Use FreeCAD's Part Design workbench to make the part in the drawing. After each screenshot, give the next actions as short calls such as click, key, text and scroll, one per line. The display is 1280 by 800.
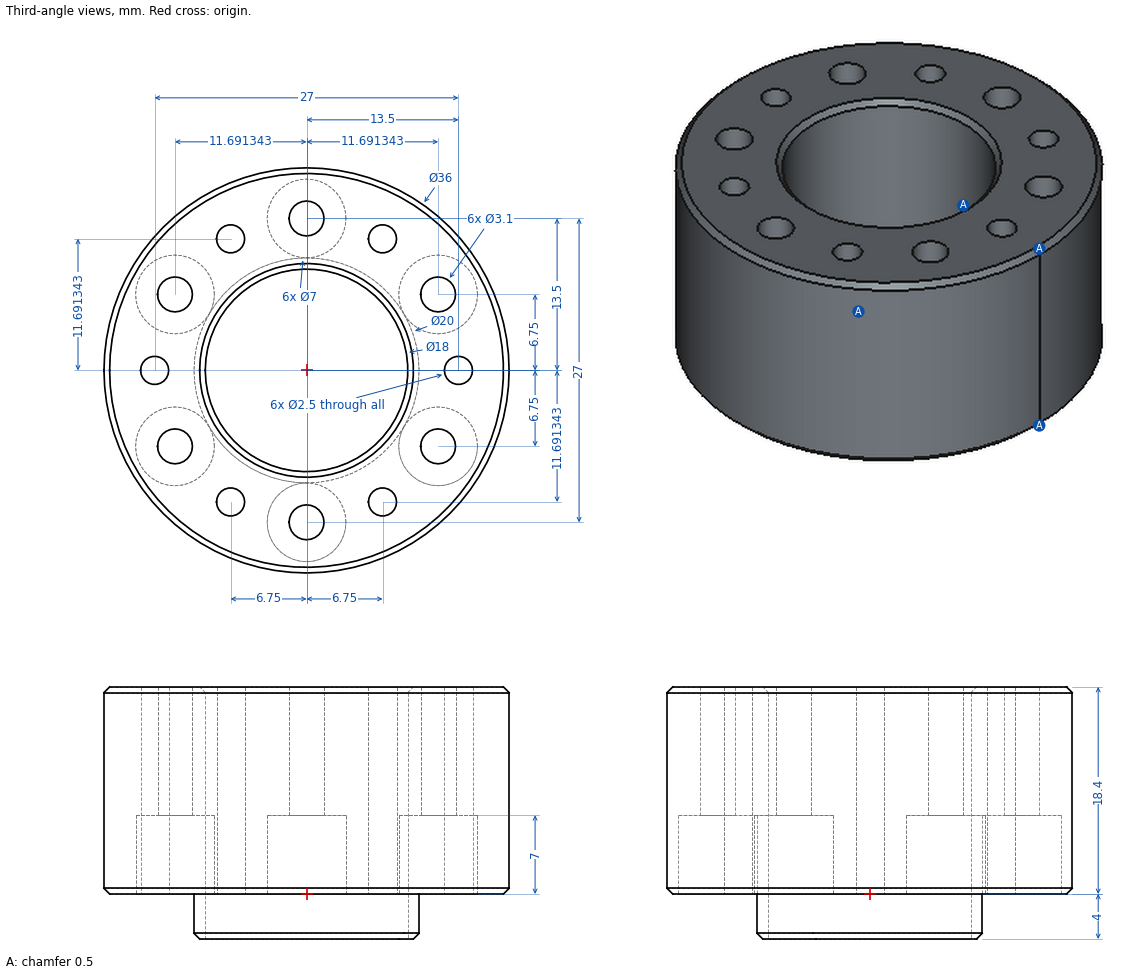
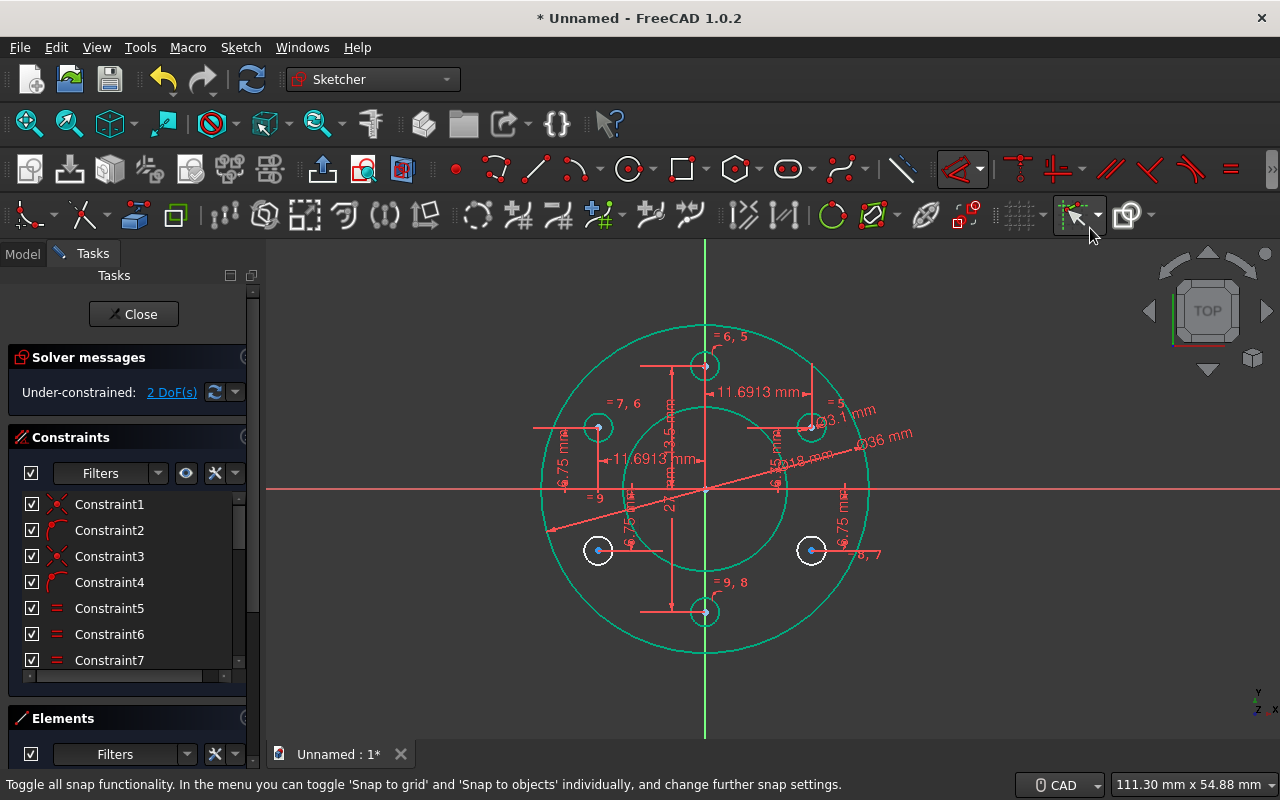
click(812, 551)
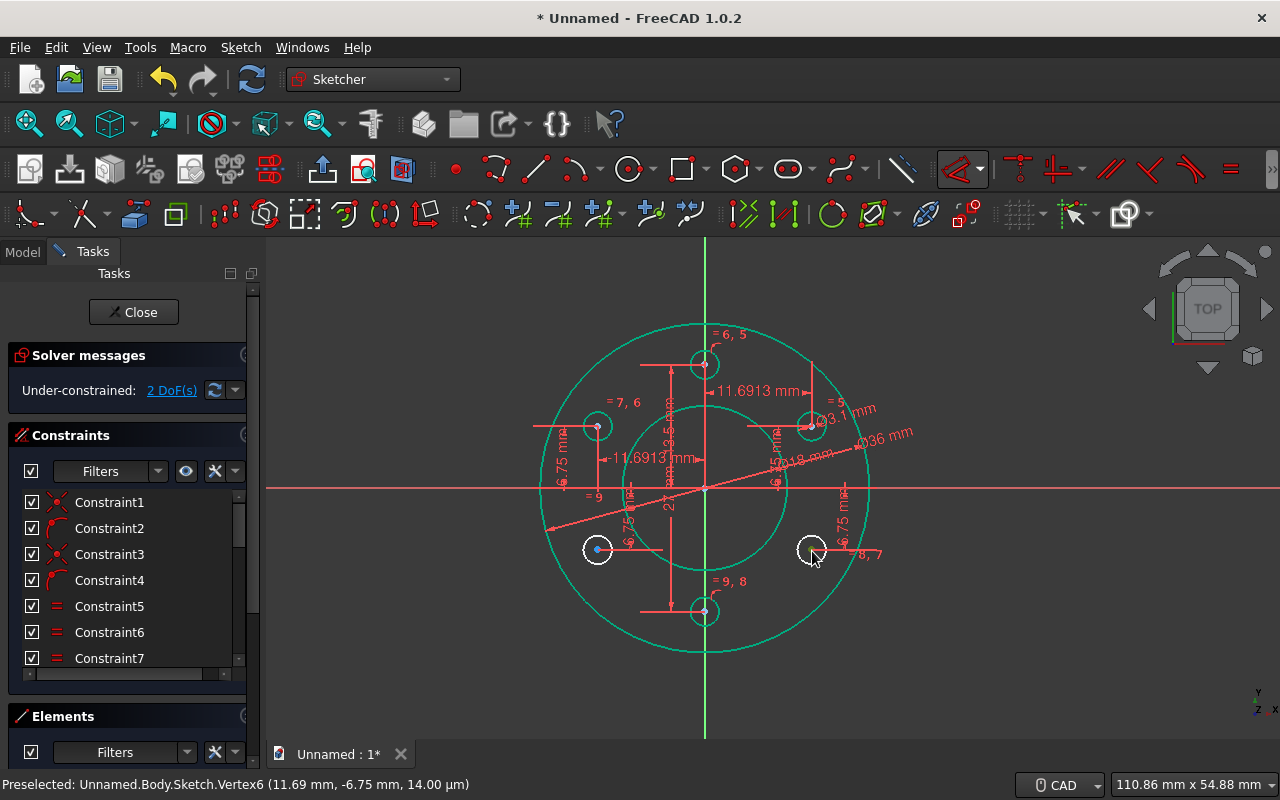
click(982, 170)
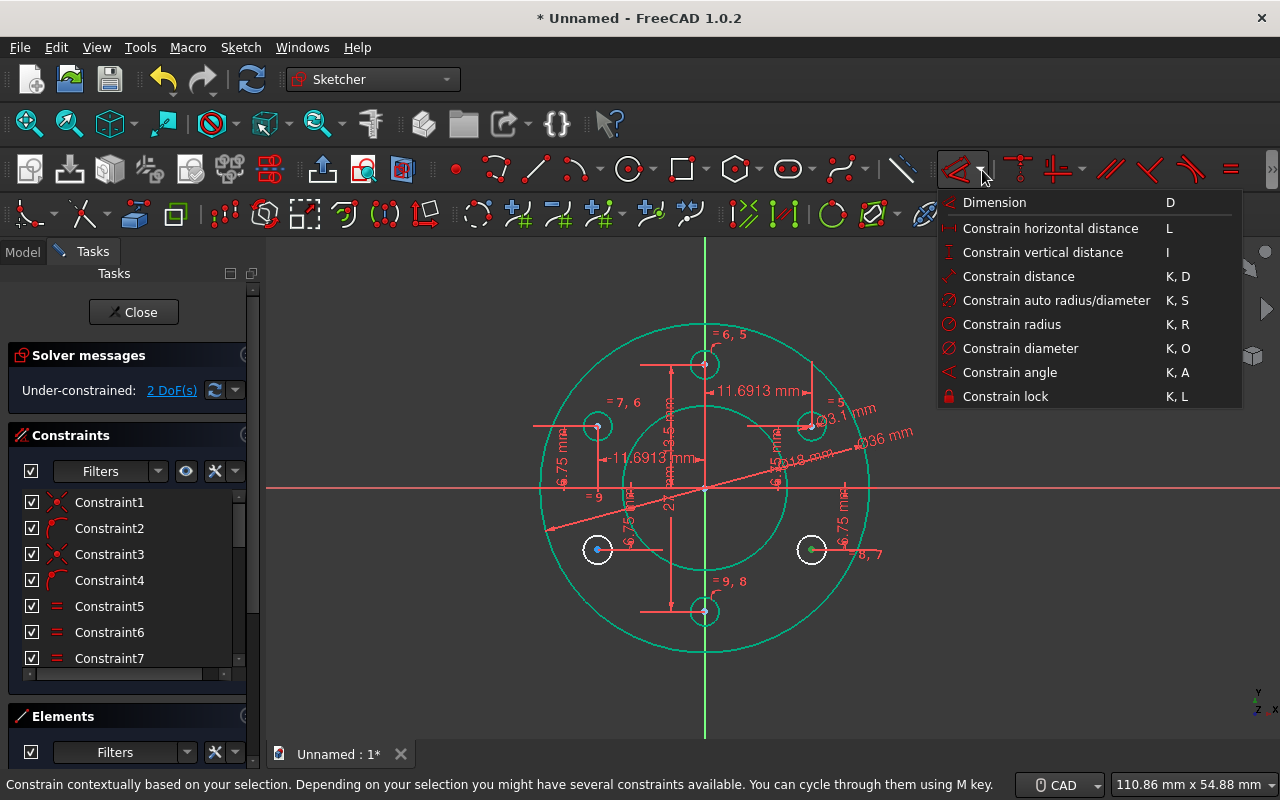
click(1090, 228)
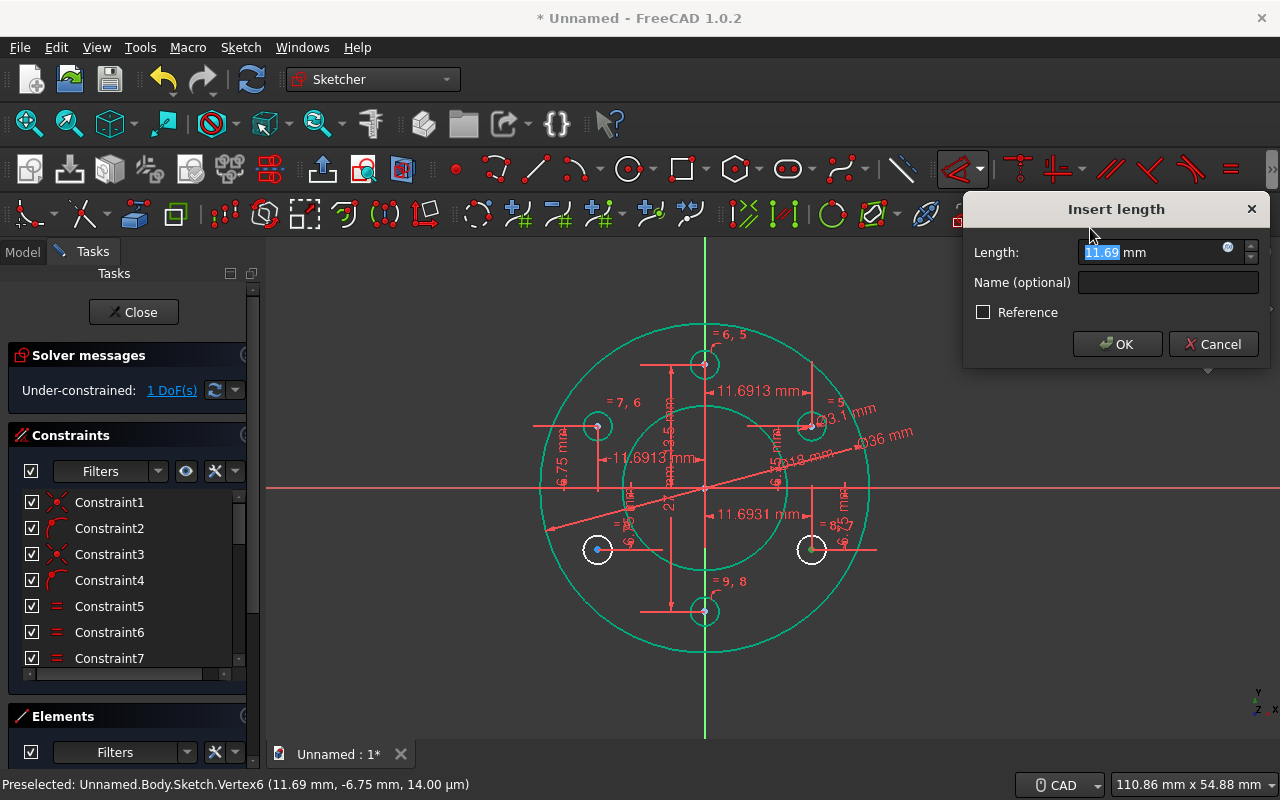
text(11.691343)
key(Return)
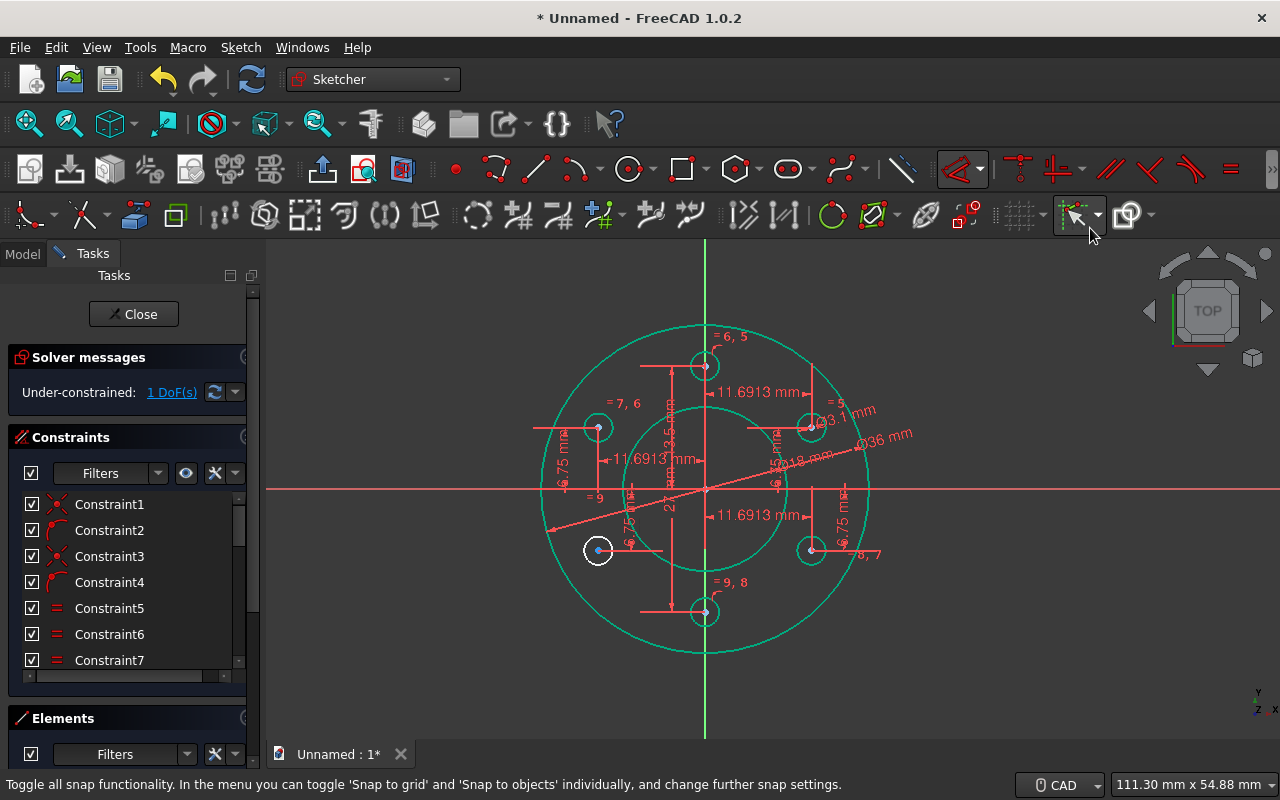
click(598, 551)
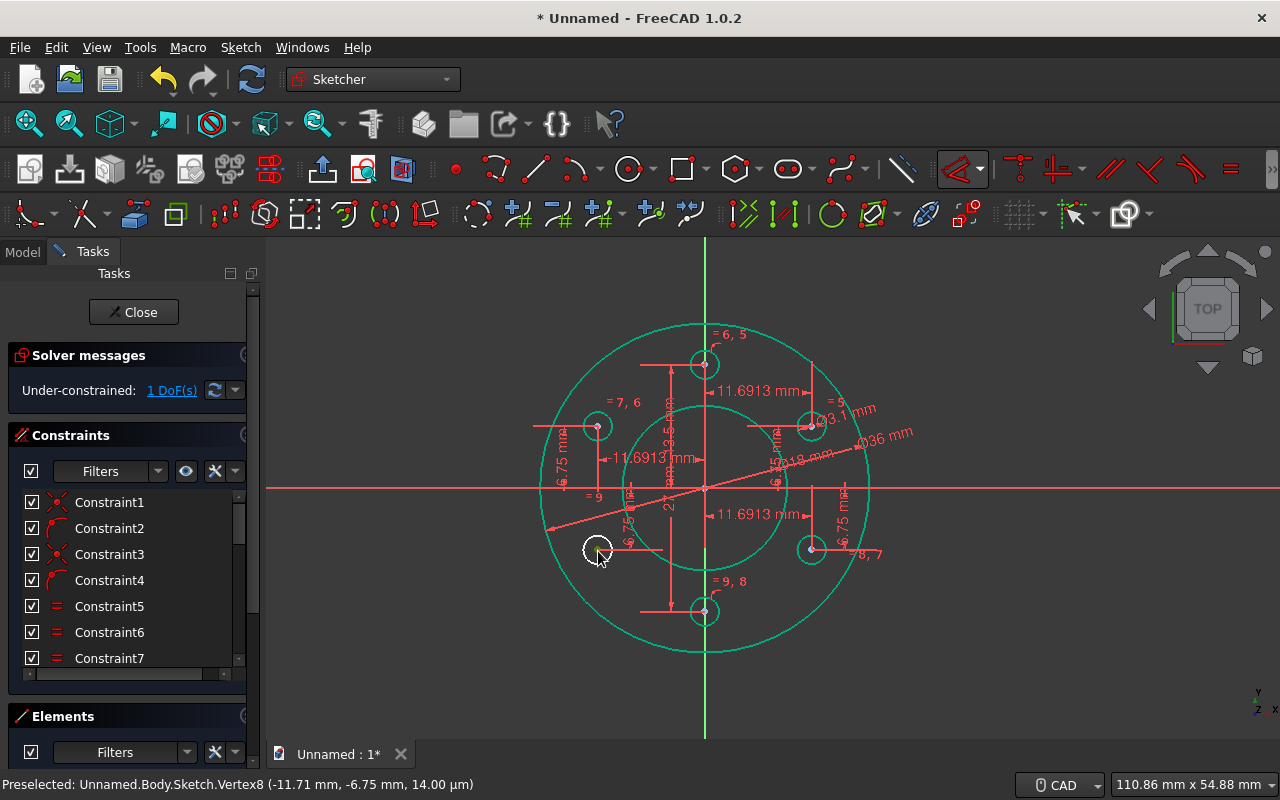
key(l)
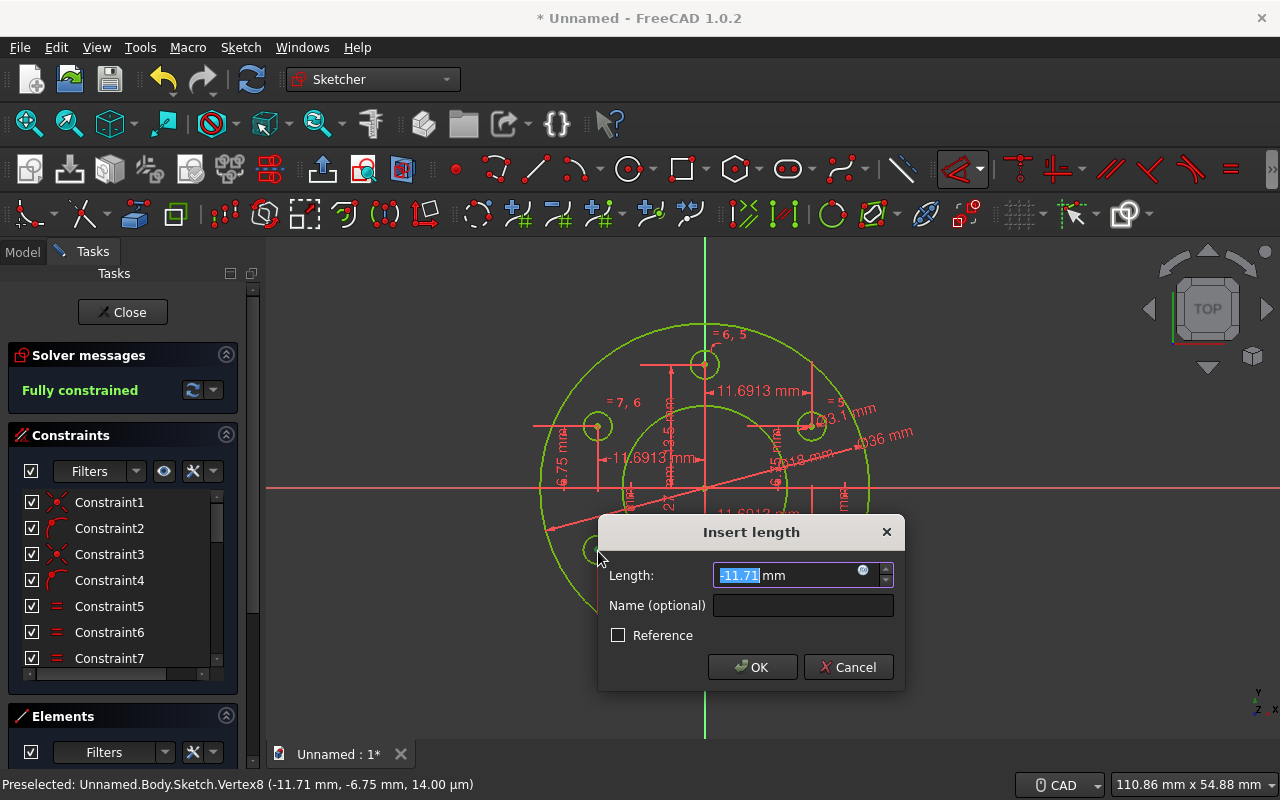
text(-11.691343)
key(Return)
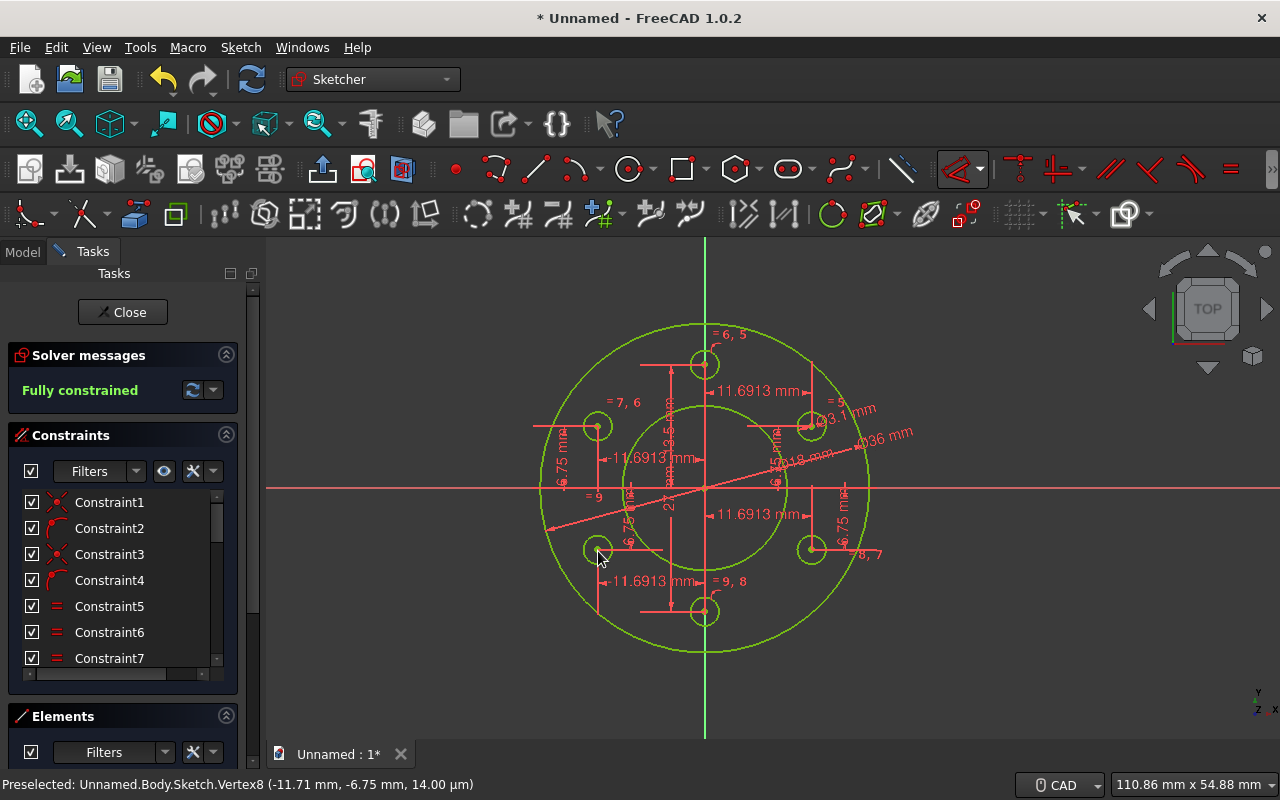
click(123, 312)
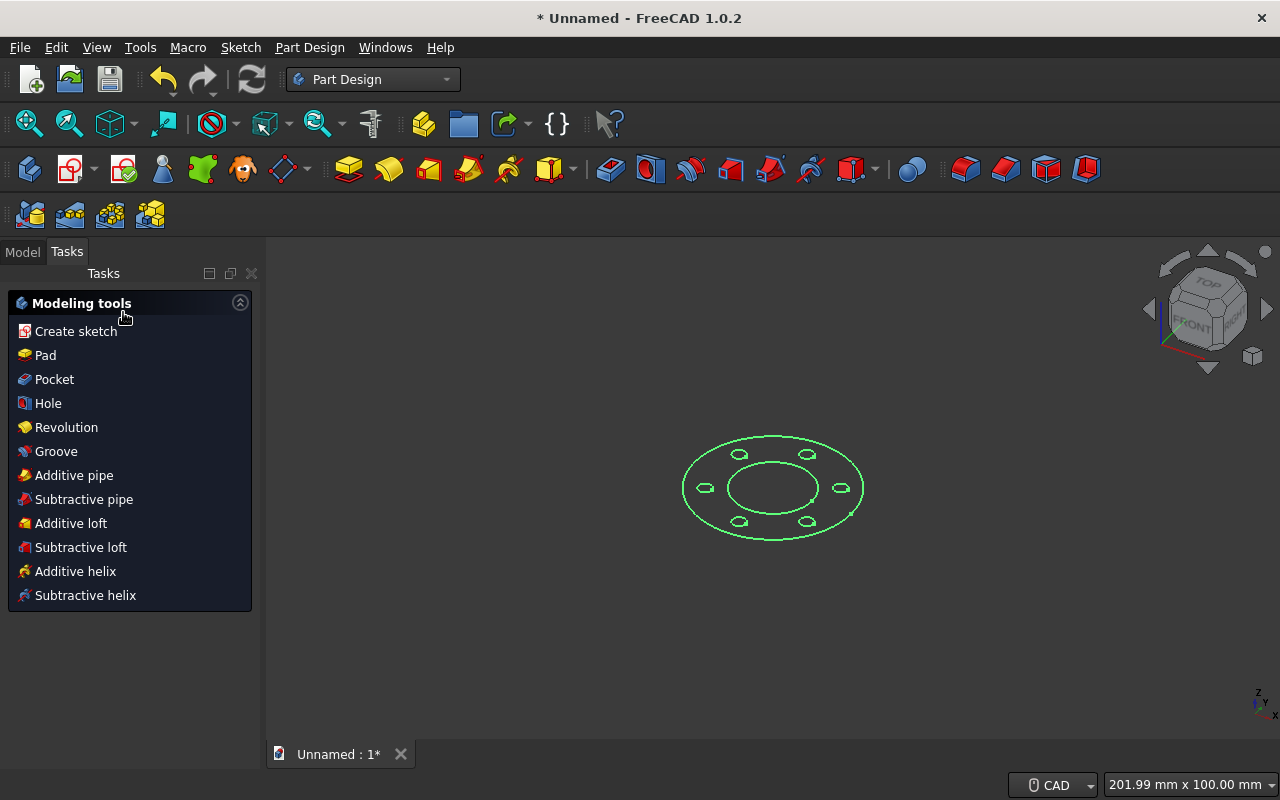
click(350, 170)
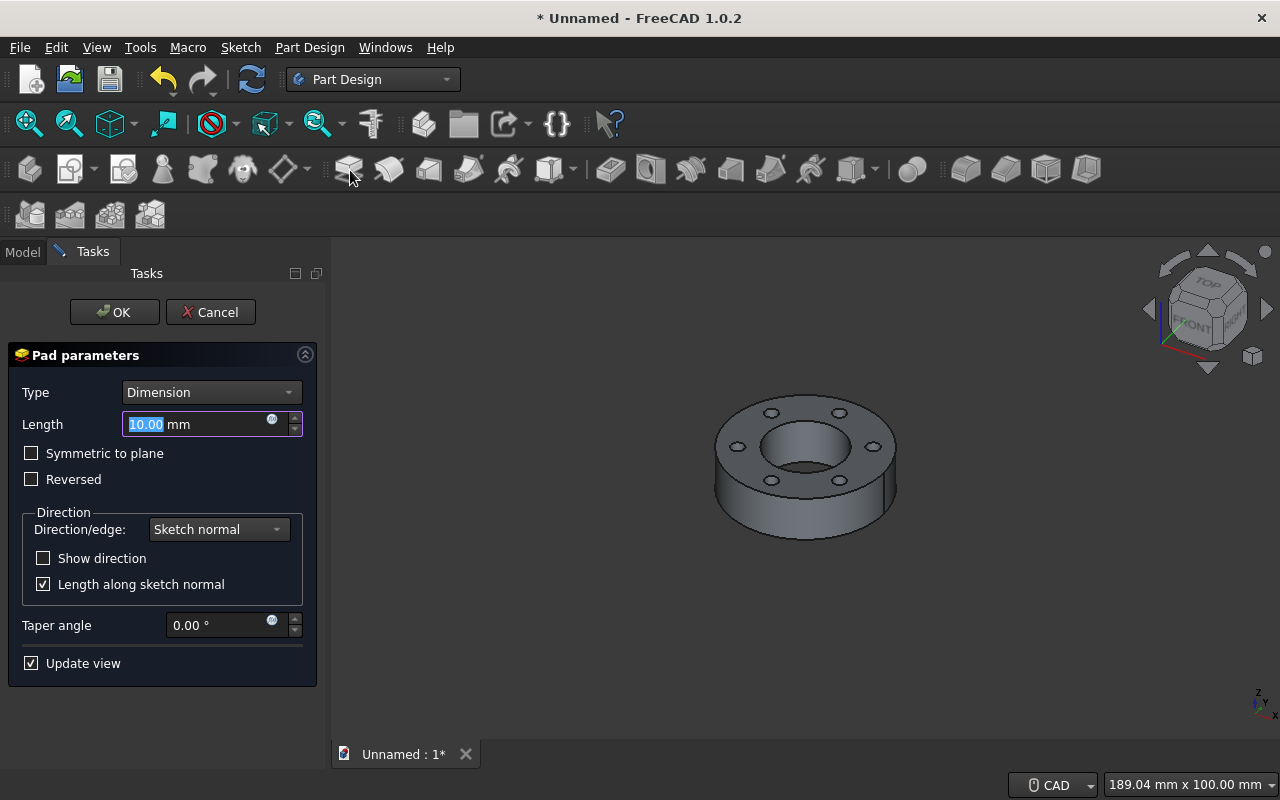
text(18.4)
key(Tab)